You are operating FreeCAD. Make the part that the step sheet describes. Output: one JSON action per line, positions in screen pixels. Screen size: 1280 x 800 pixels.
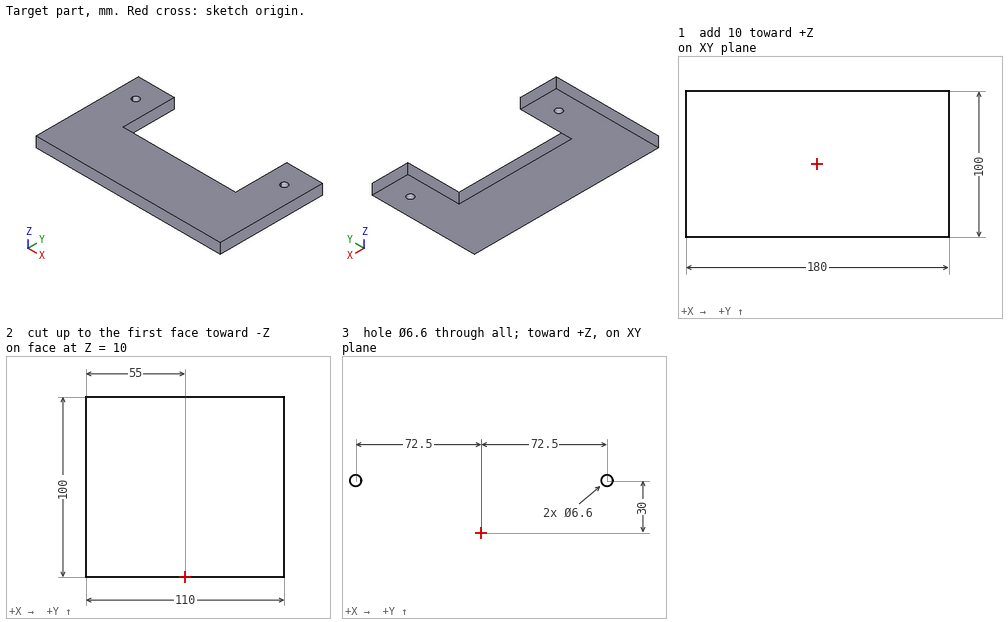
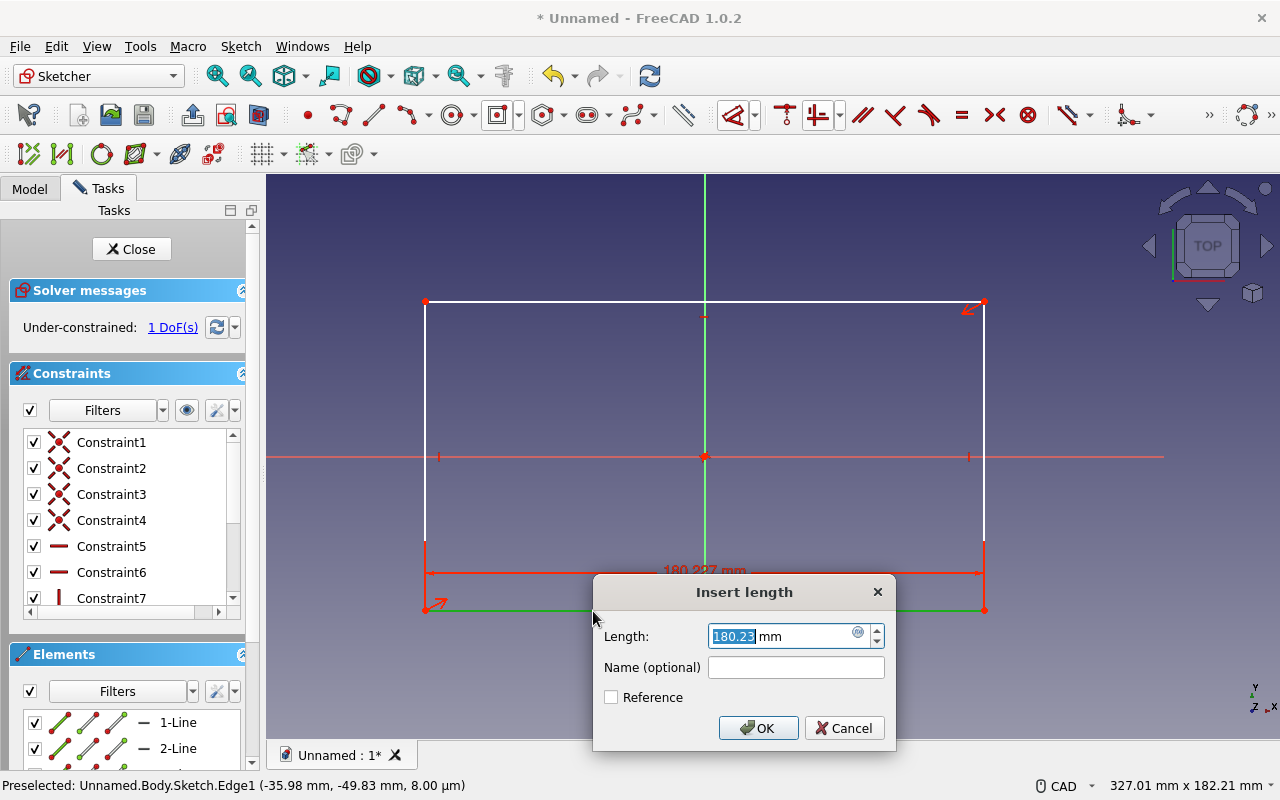
{"action": "type", "text": "180"}
{"action": "key", "text": "Return"}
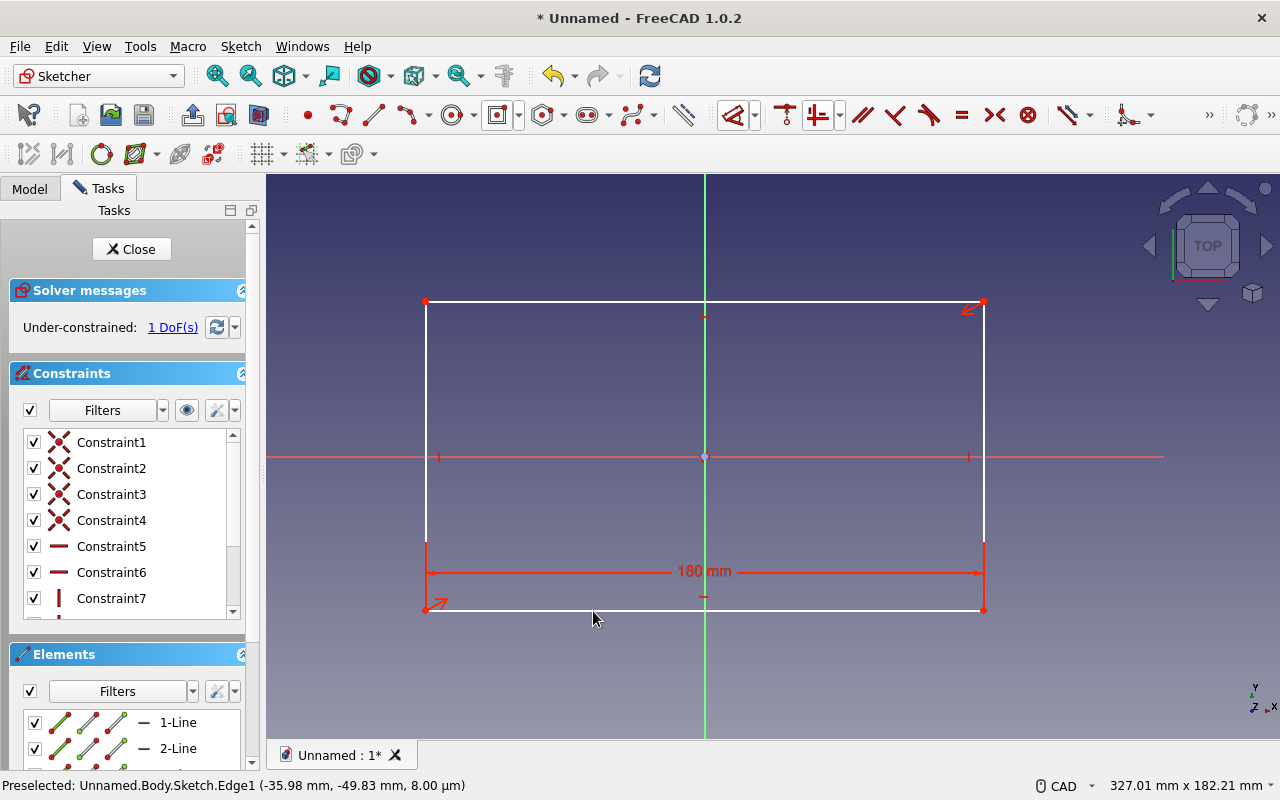
{"action": "left_click", "coordinate": [984, 518]}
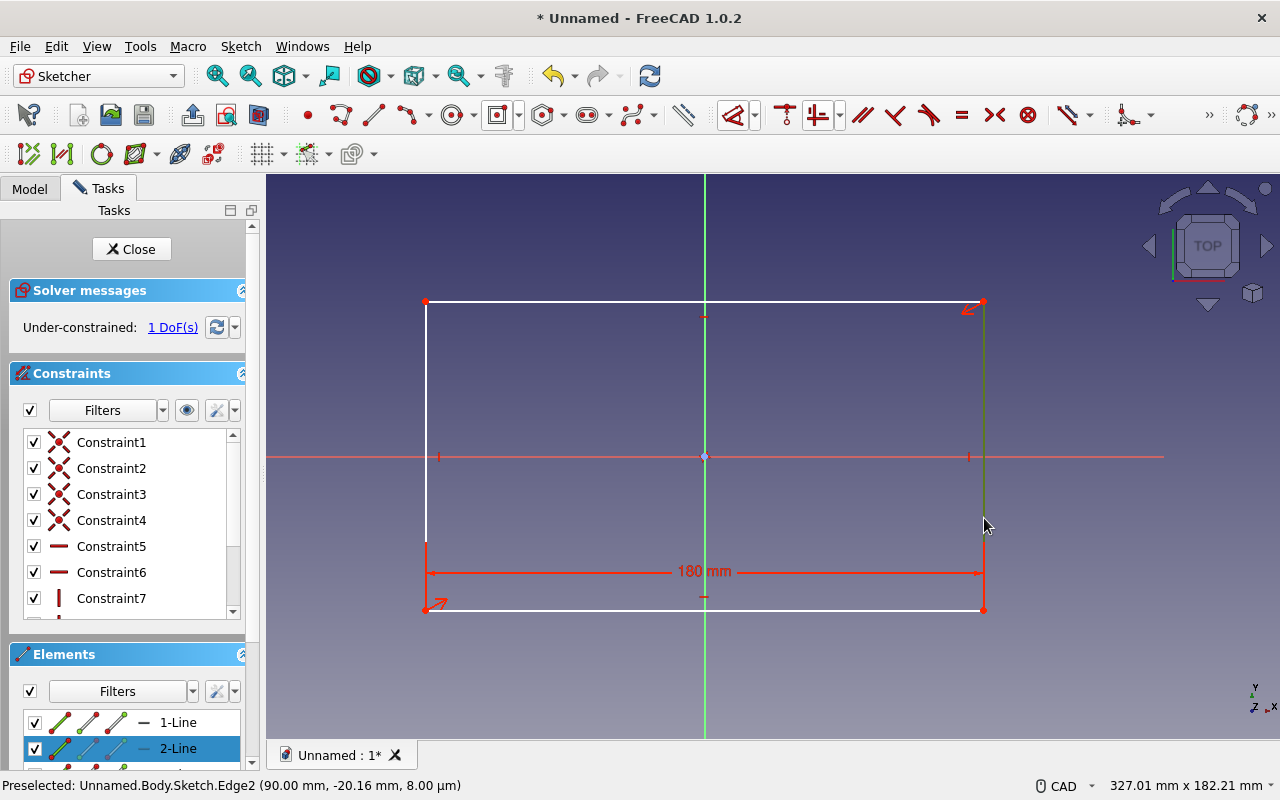
{"action": "key", "text": "i"}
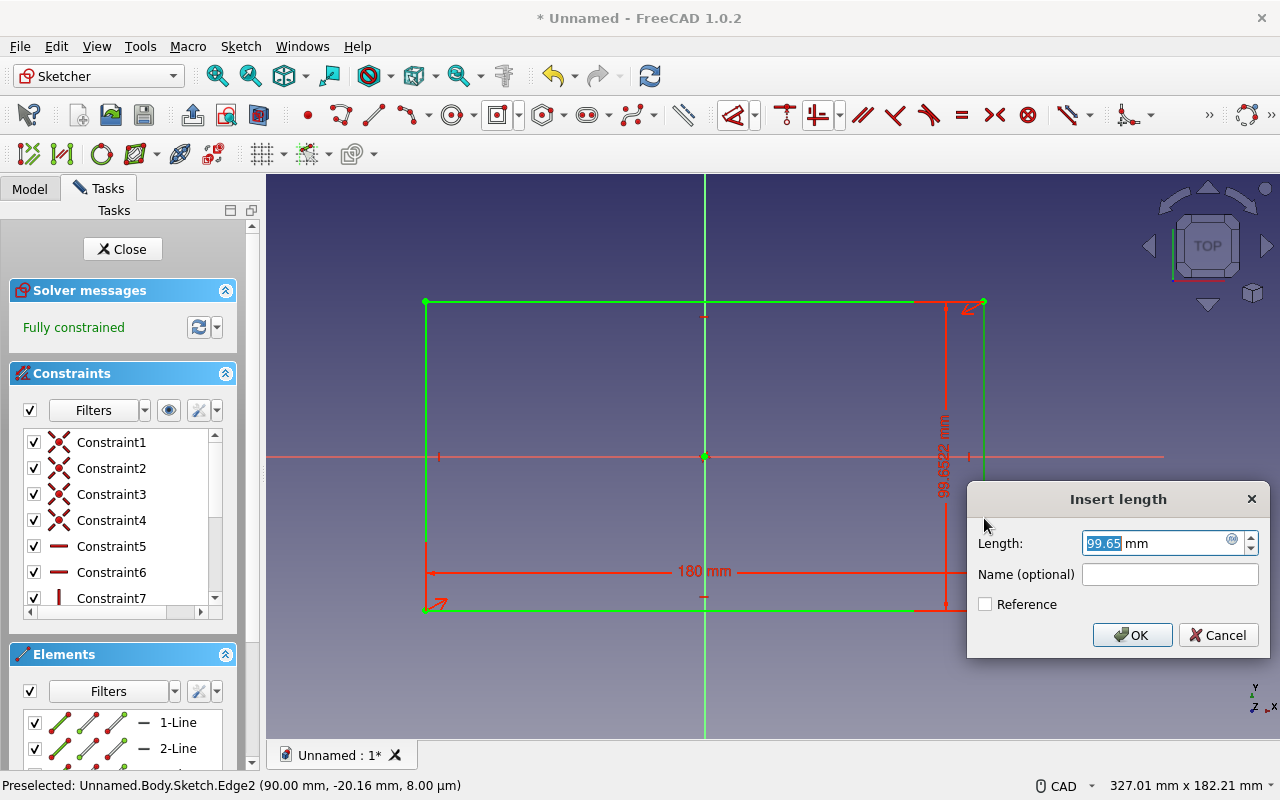
{"action": "type", "text": "100"}
{"action": "key", "text": "Return"}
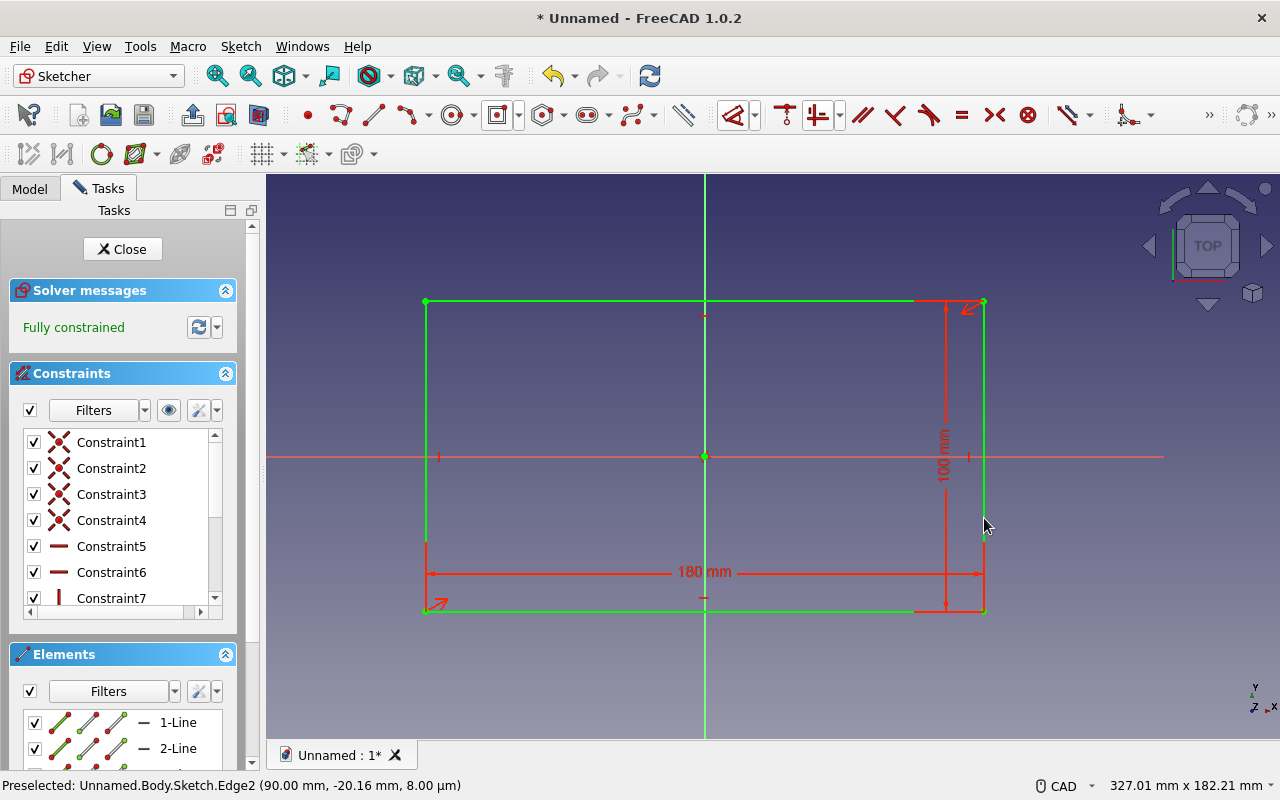
{"action": "left_click", "coordinate": [123, 249]}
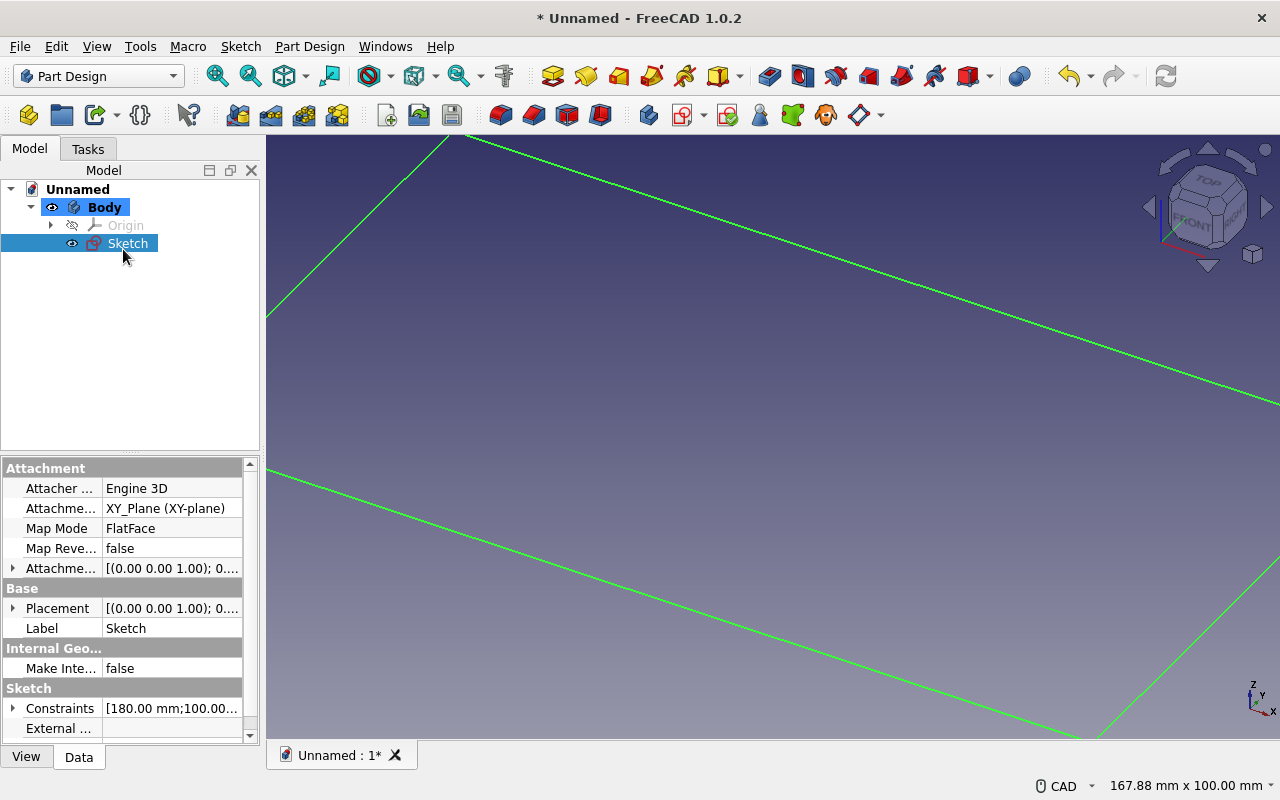
{"action": "left_click", "coordinate": [553, 76]}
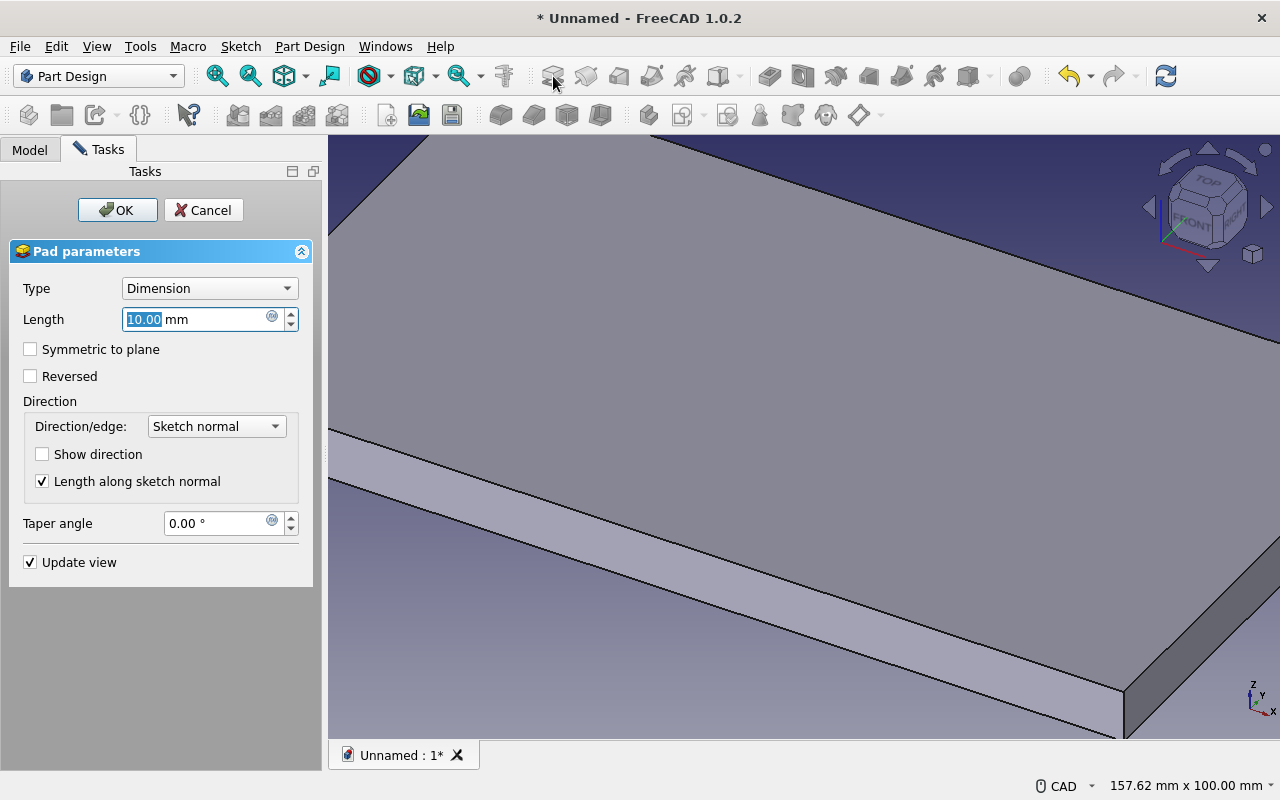
{"action": "type", "text": "10"}
{"action": "key", "text": "Tab"}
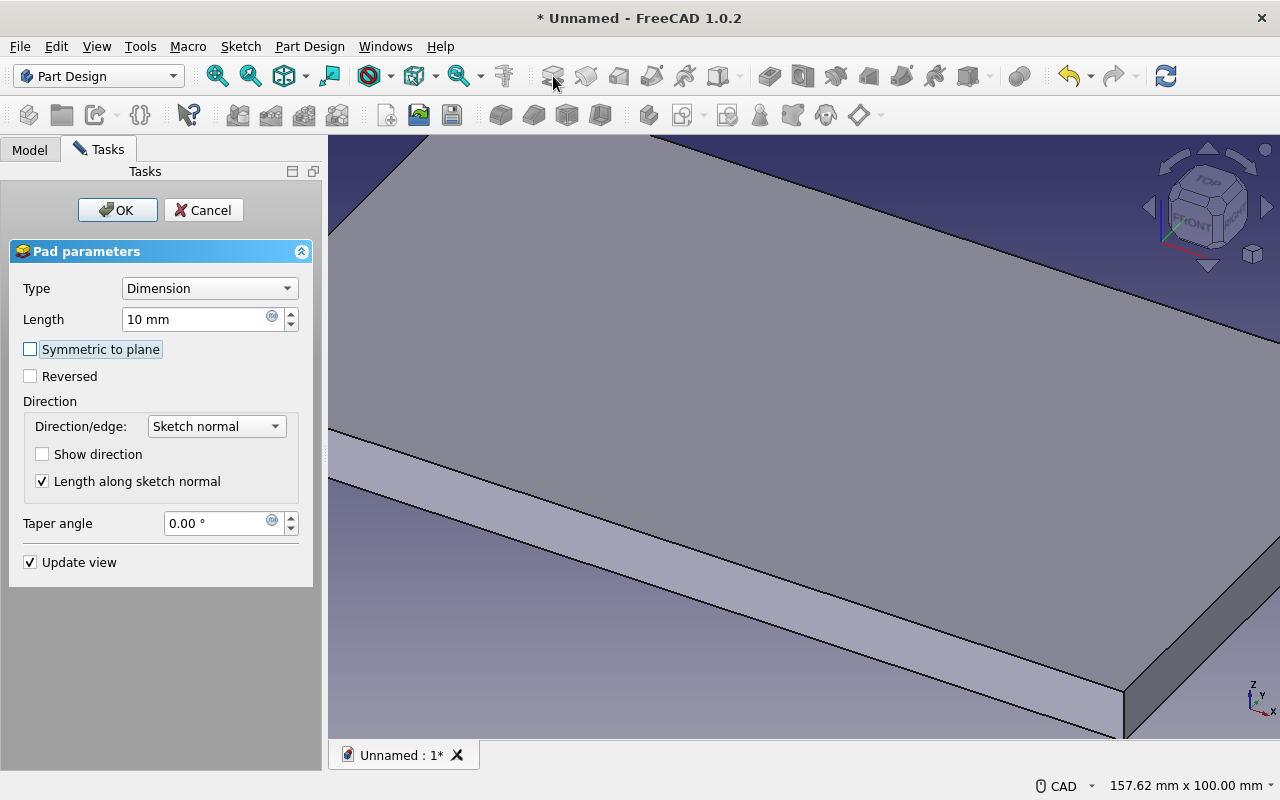
{"action": "left_click", "coordinate": [118, 210]}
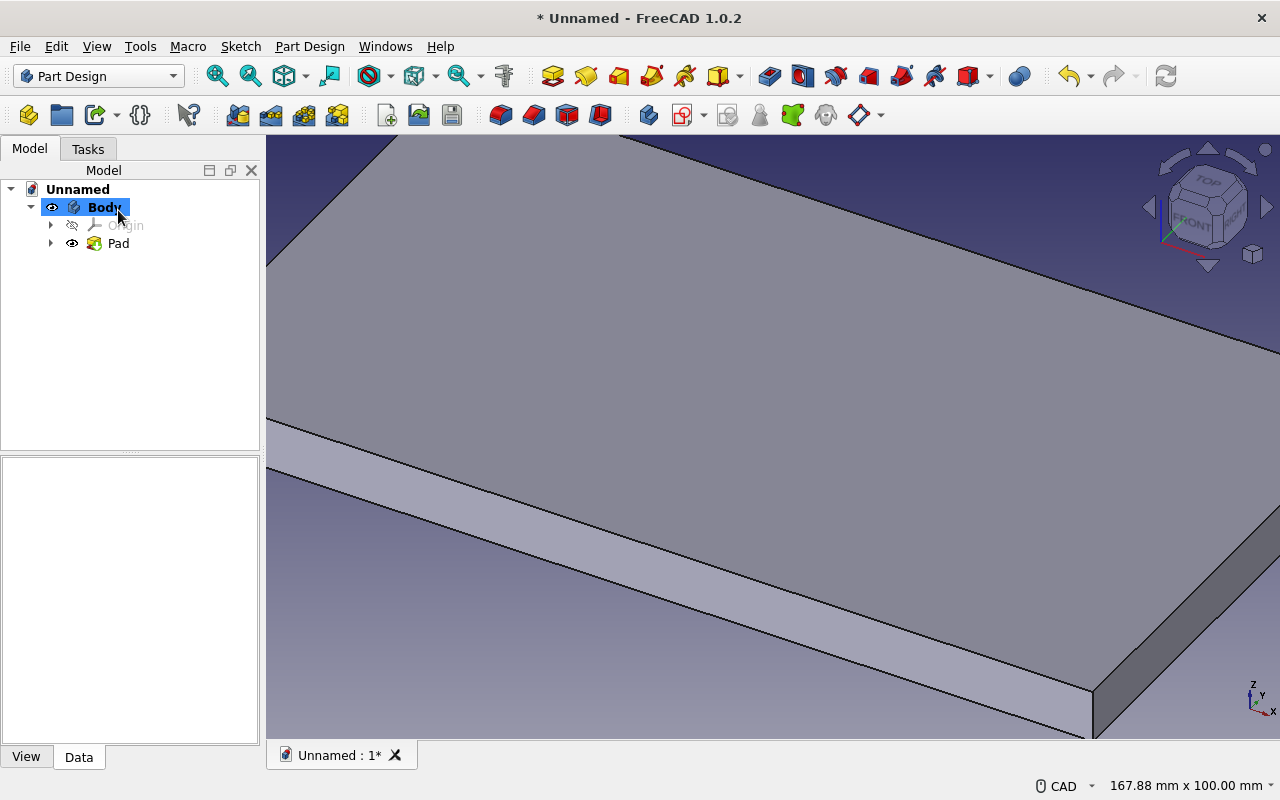
{"action": "left_click", "coordinate": [218, 76]}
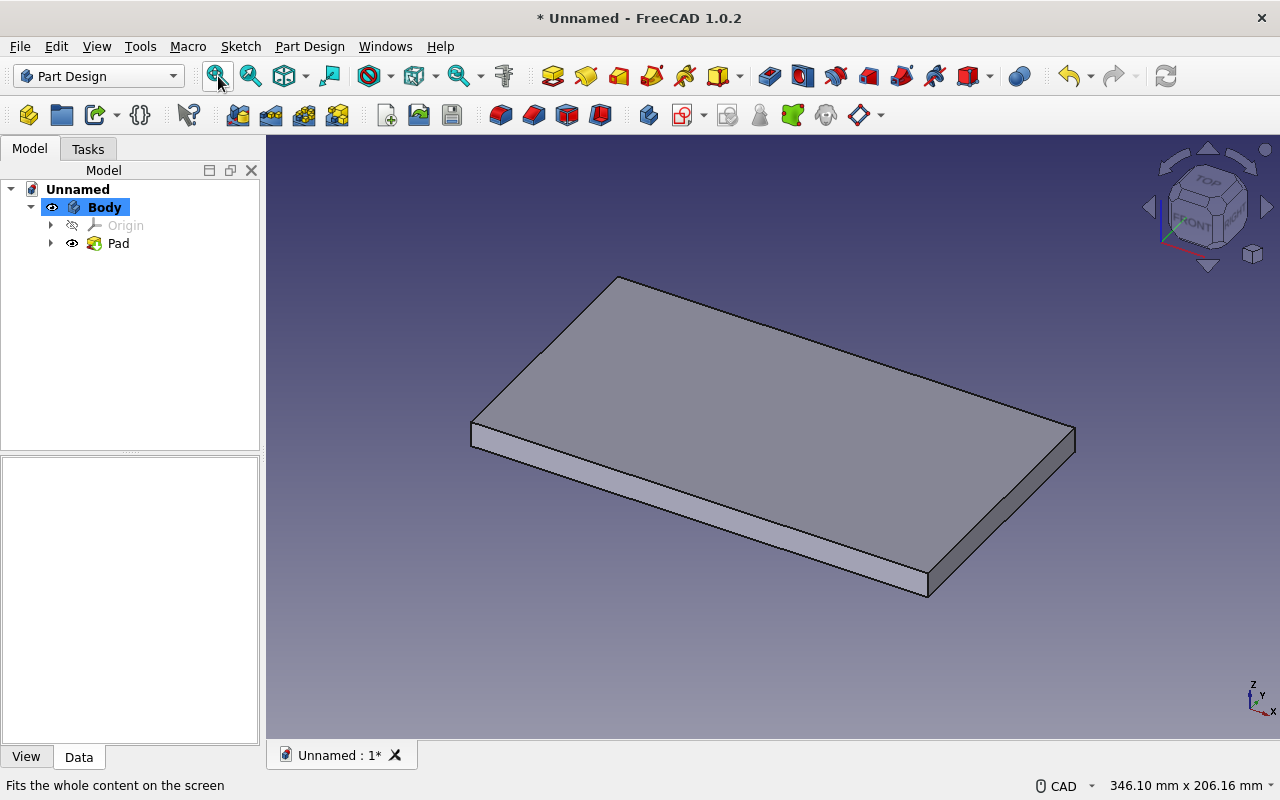
{"action": "left_click", "coordinate": [838, 446]}